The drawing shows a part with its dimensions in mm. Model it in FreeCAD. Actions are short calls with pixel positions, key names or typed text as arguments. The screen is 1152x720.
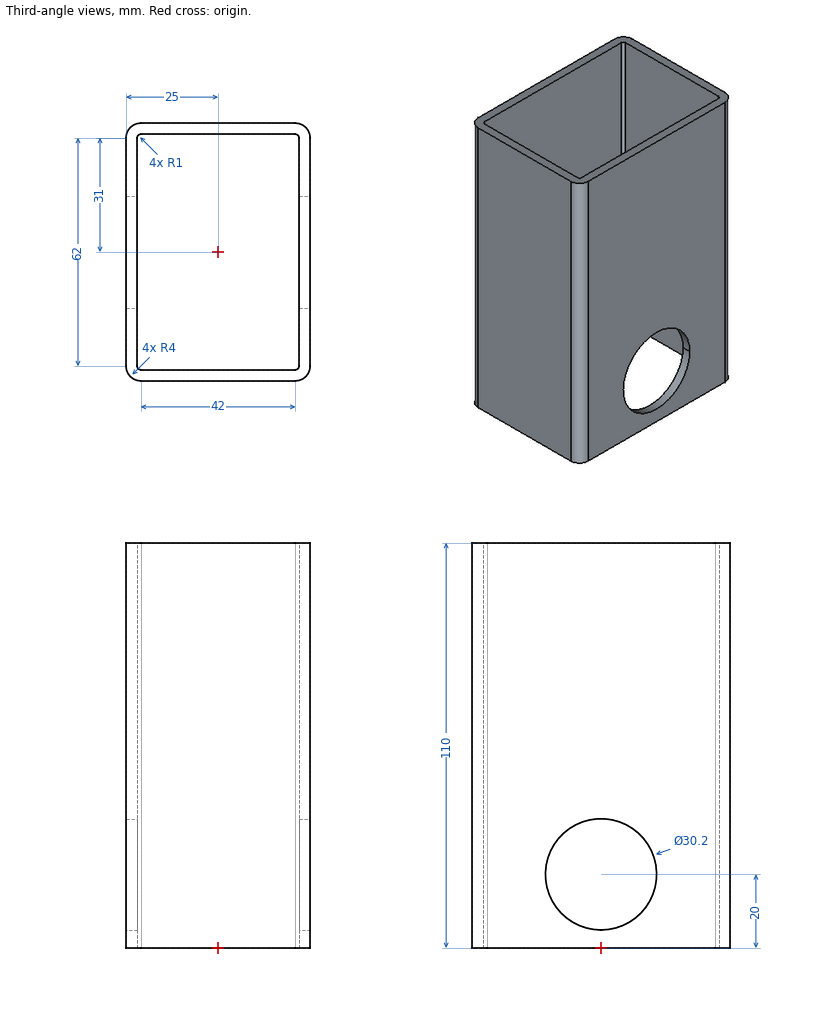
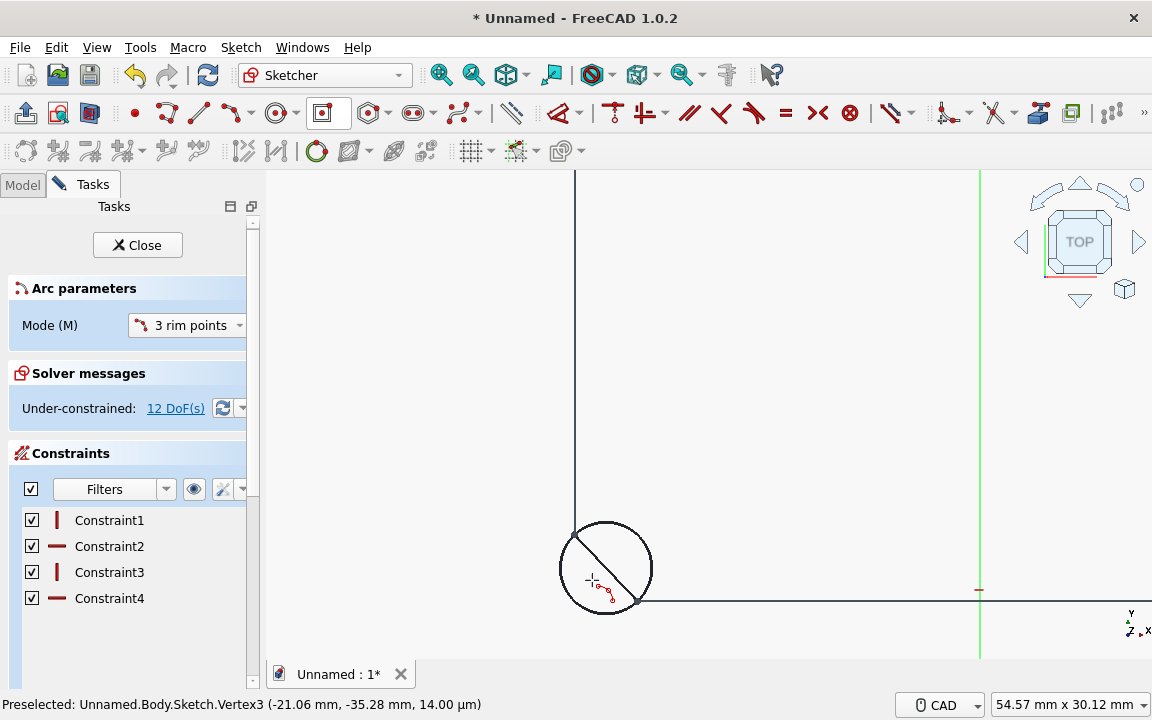
click(593, 578)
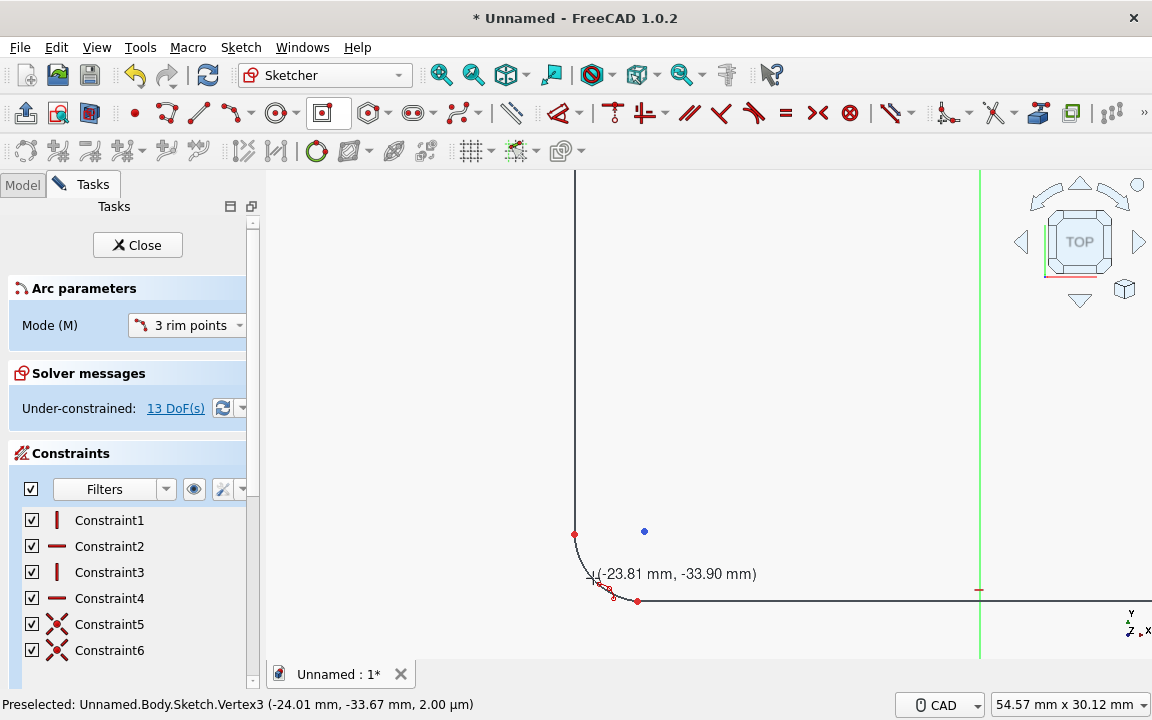
scroll(530, 541, down, 7)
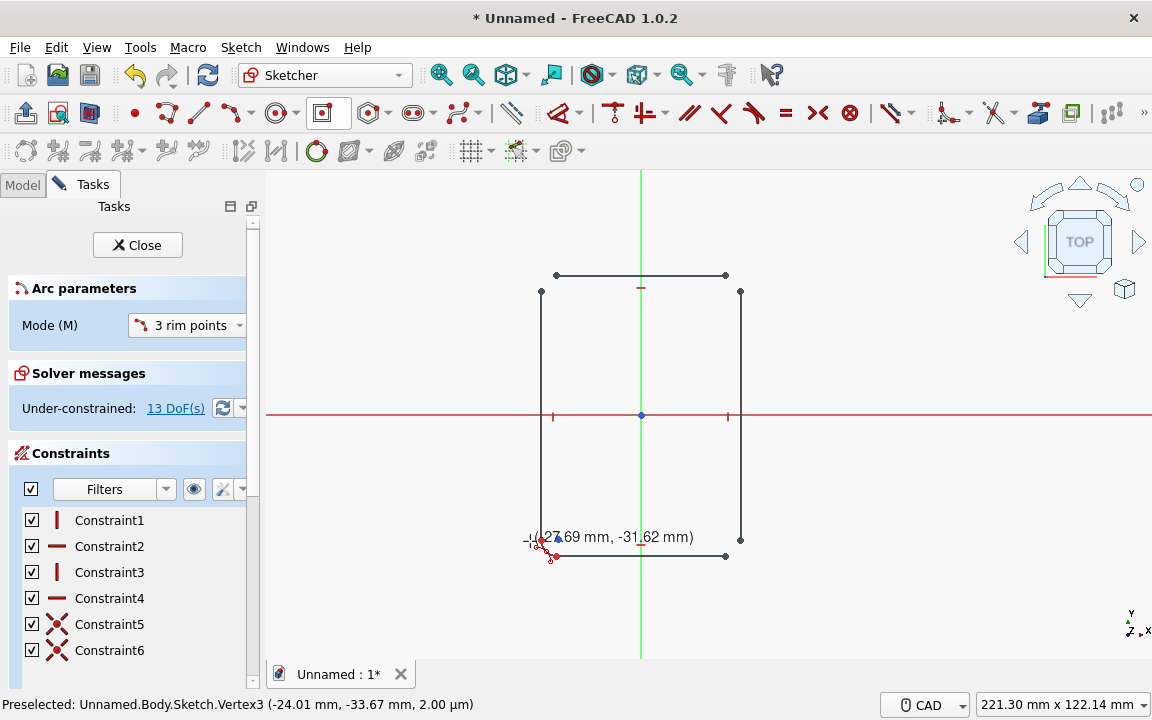
click(725, 556)
click(741, 540)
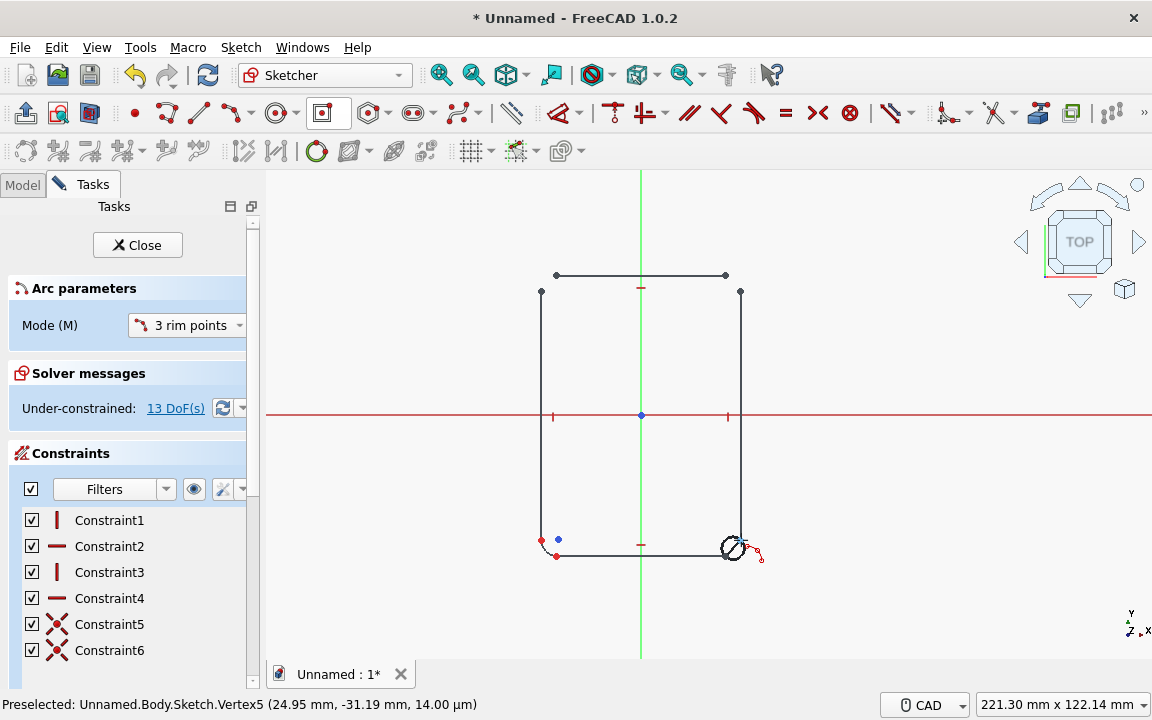
scroll(736, 551, up, 7)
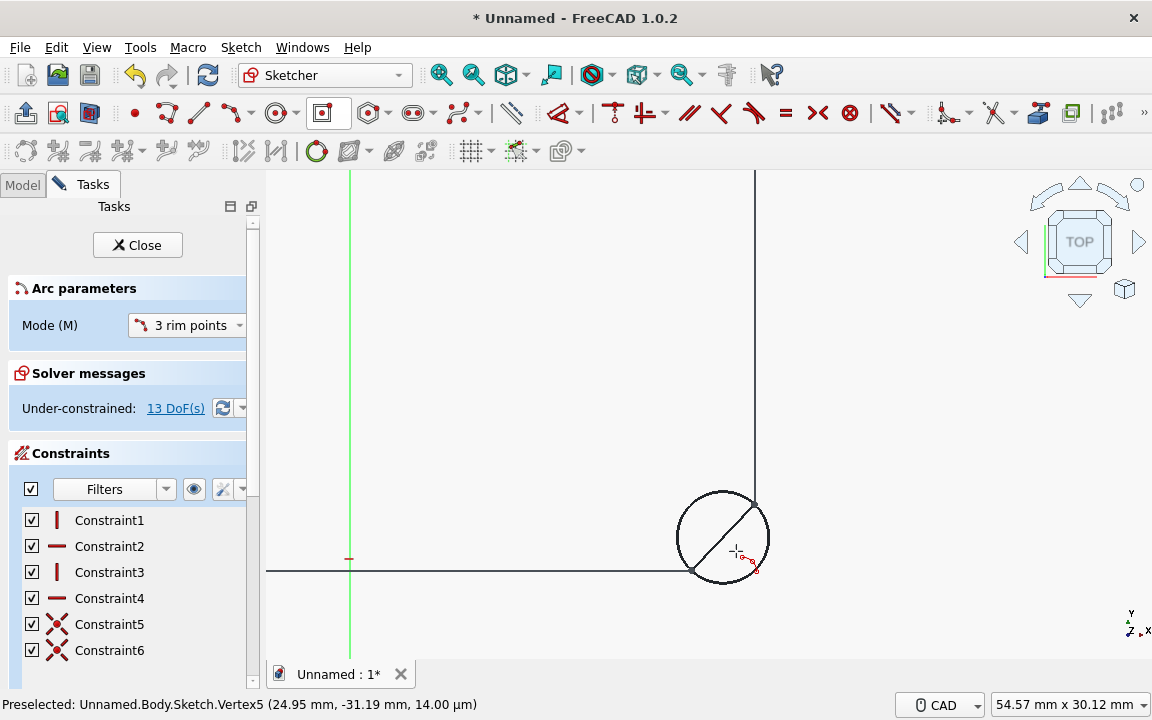
click(736, 547)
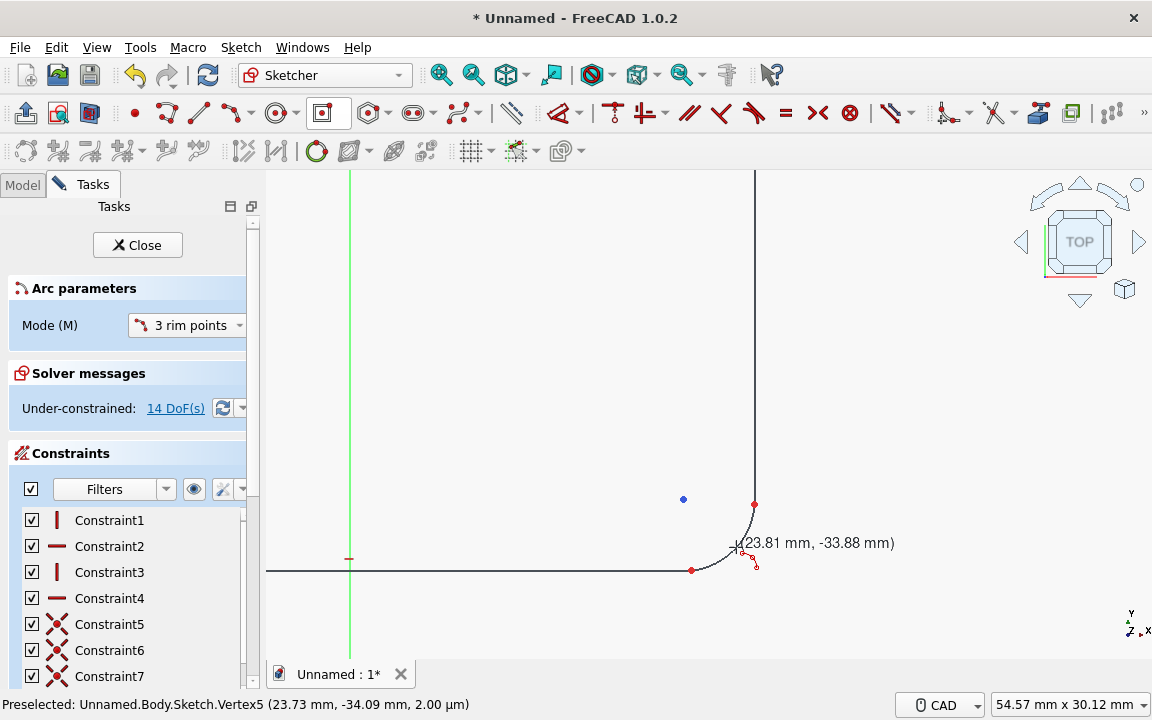
scroll(736, 551, down, 7)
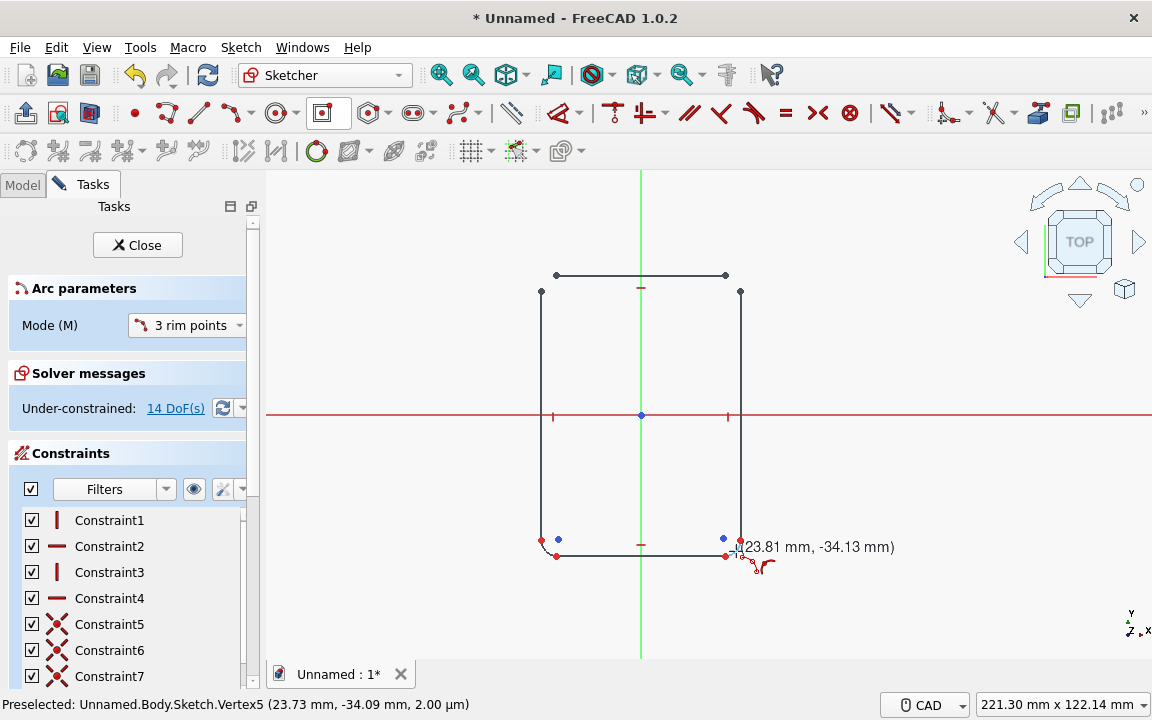
click(741, 292)
click(725, 276)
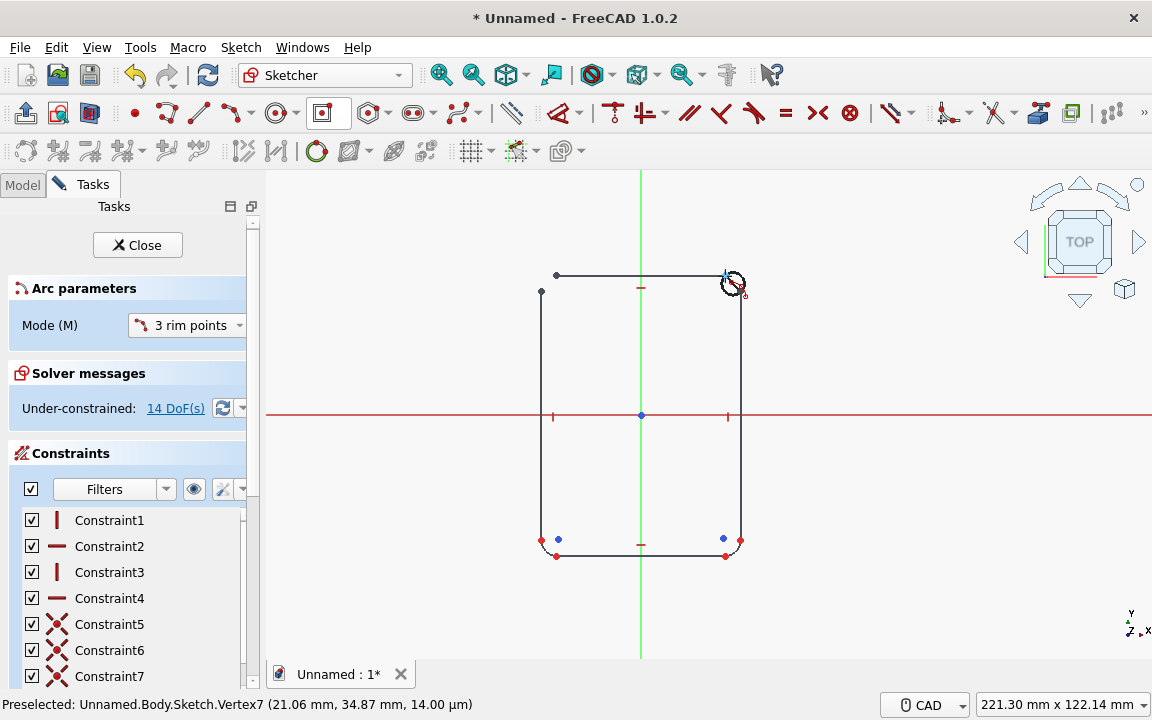
scroll(736, 280, up, 7)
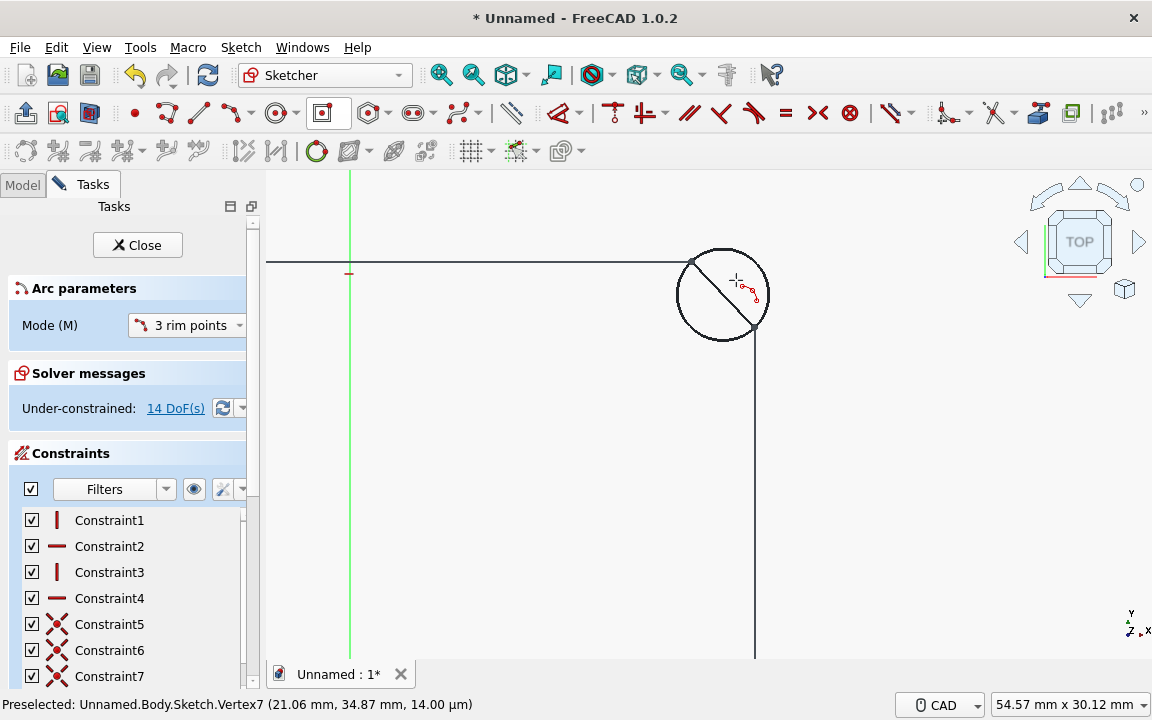
click(736, 278)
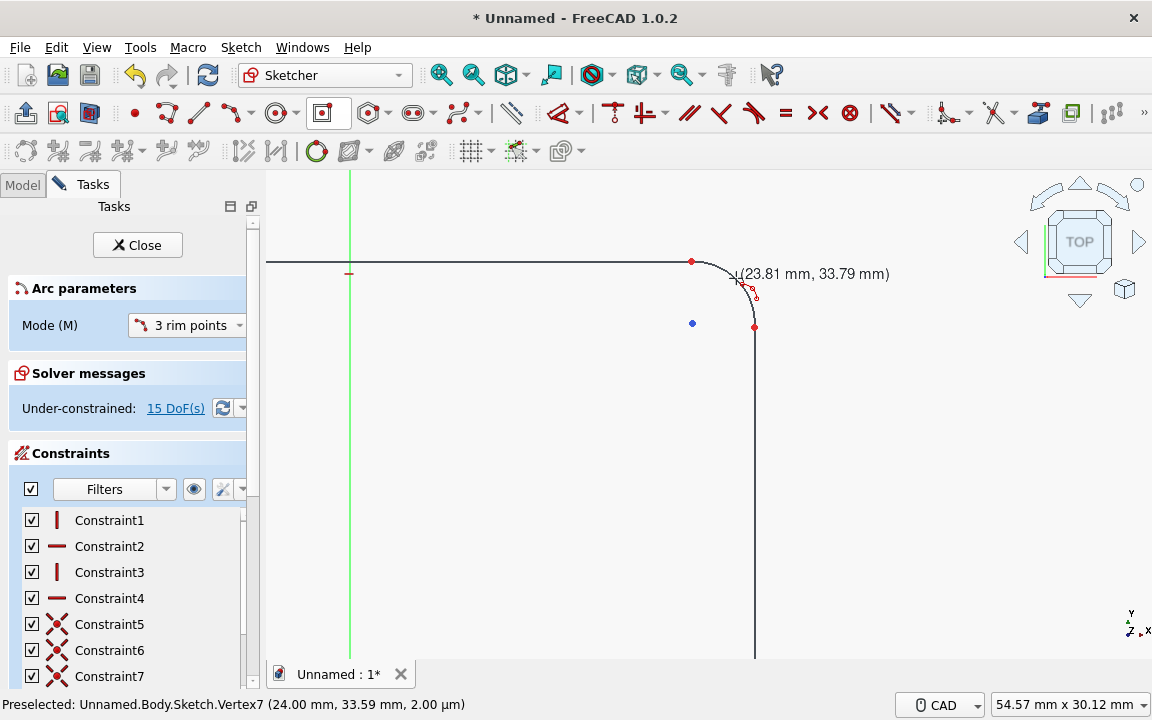
scroll(736, 279, down, 7)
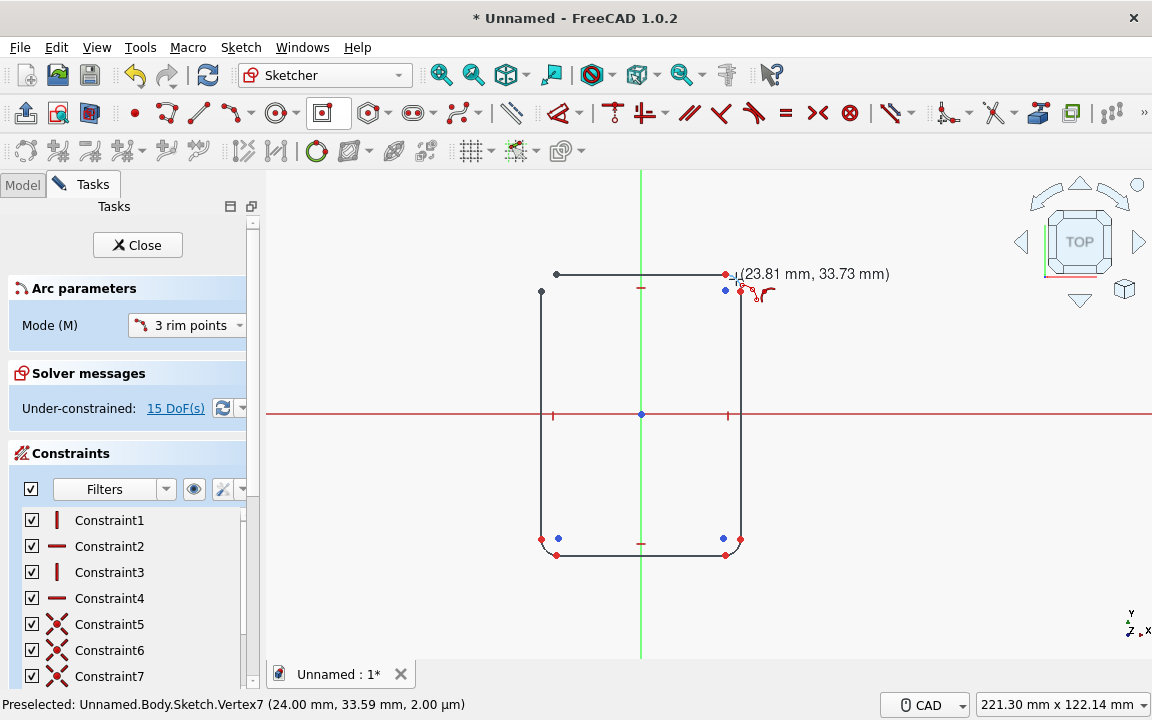
click(557, 275)
click(541, 291)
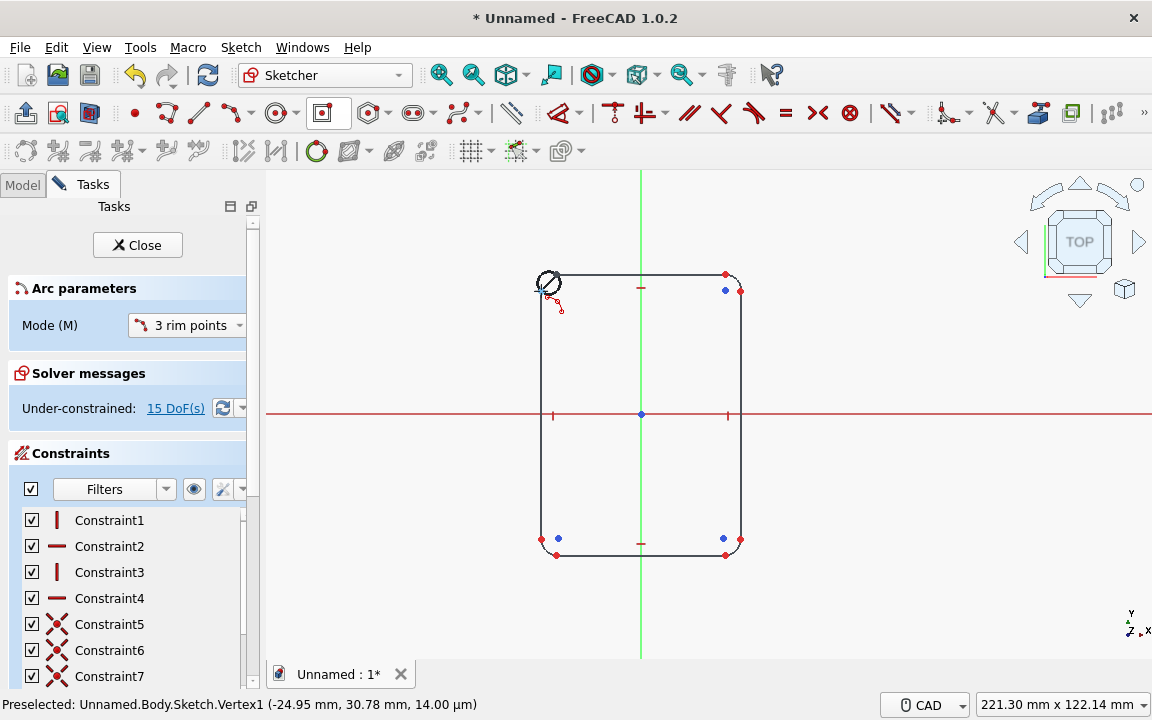
scroll(546, 279, up, 7)